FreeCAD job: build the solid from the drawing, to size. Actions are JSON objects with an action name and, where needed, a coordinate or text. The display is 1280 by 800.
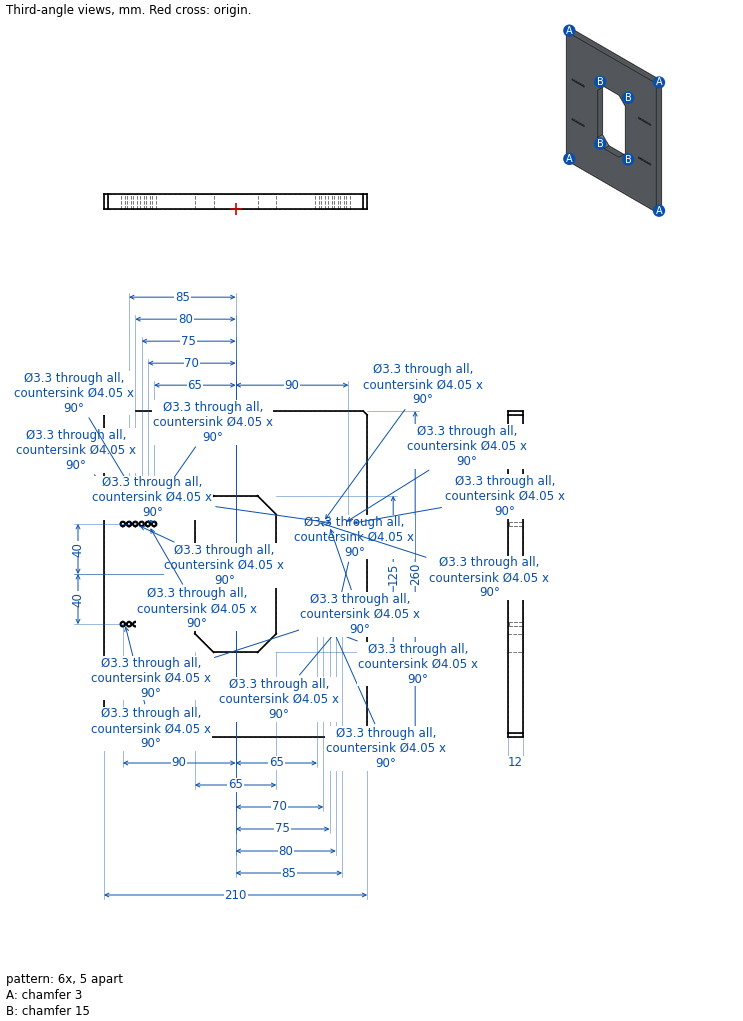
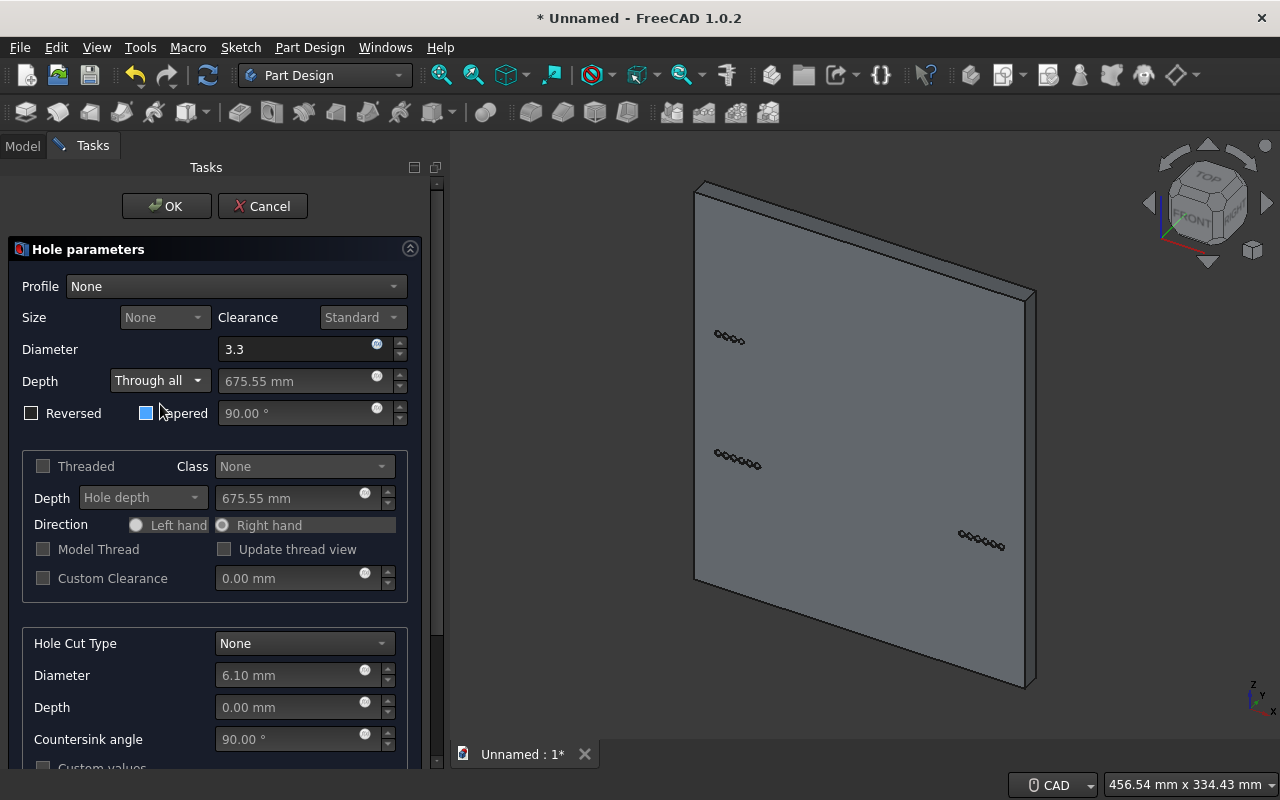
{"action": "left_click", "coordinate": [306, 644]}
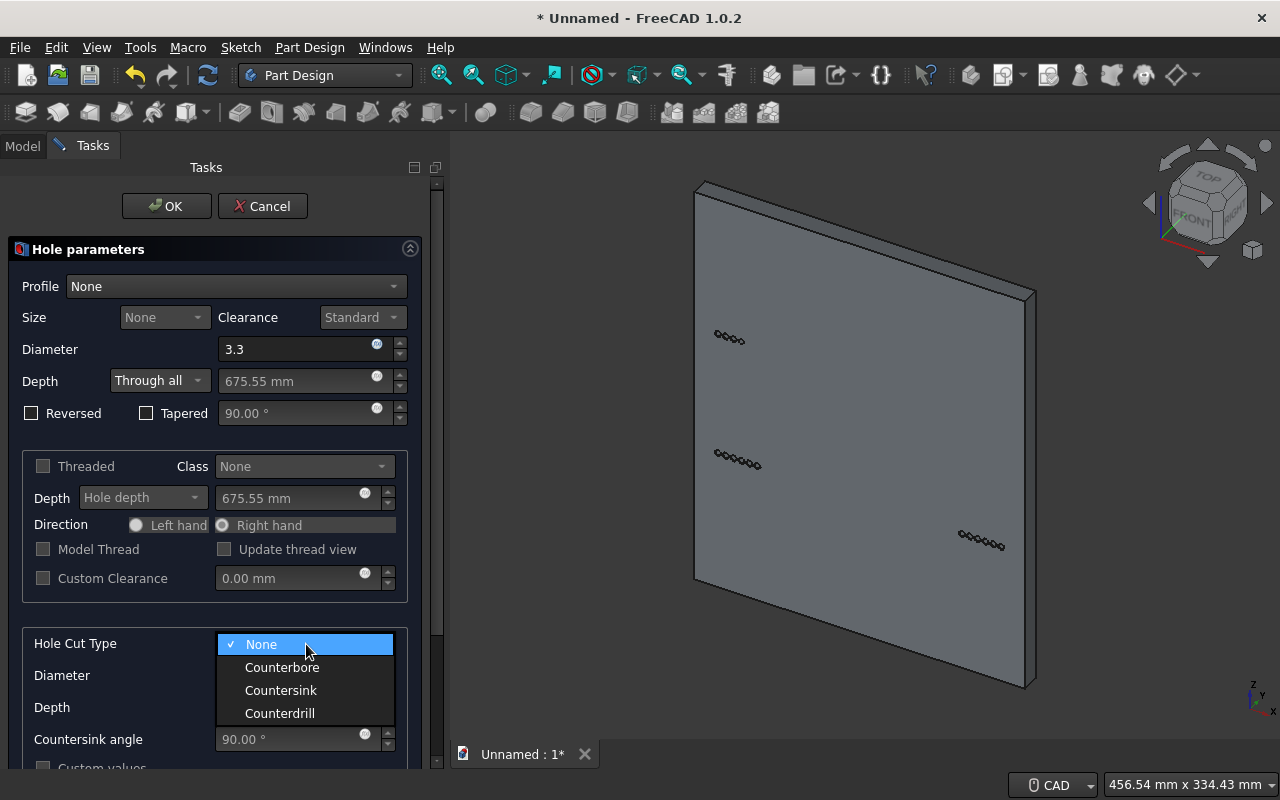
{"action": "left_click", "coordinate": [304, 690]}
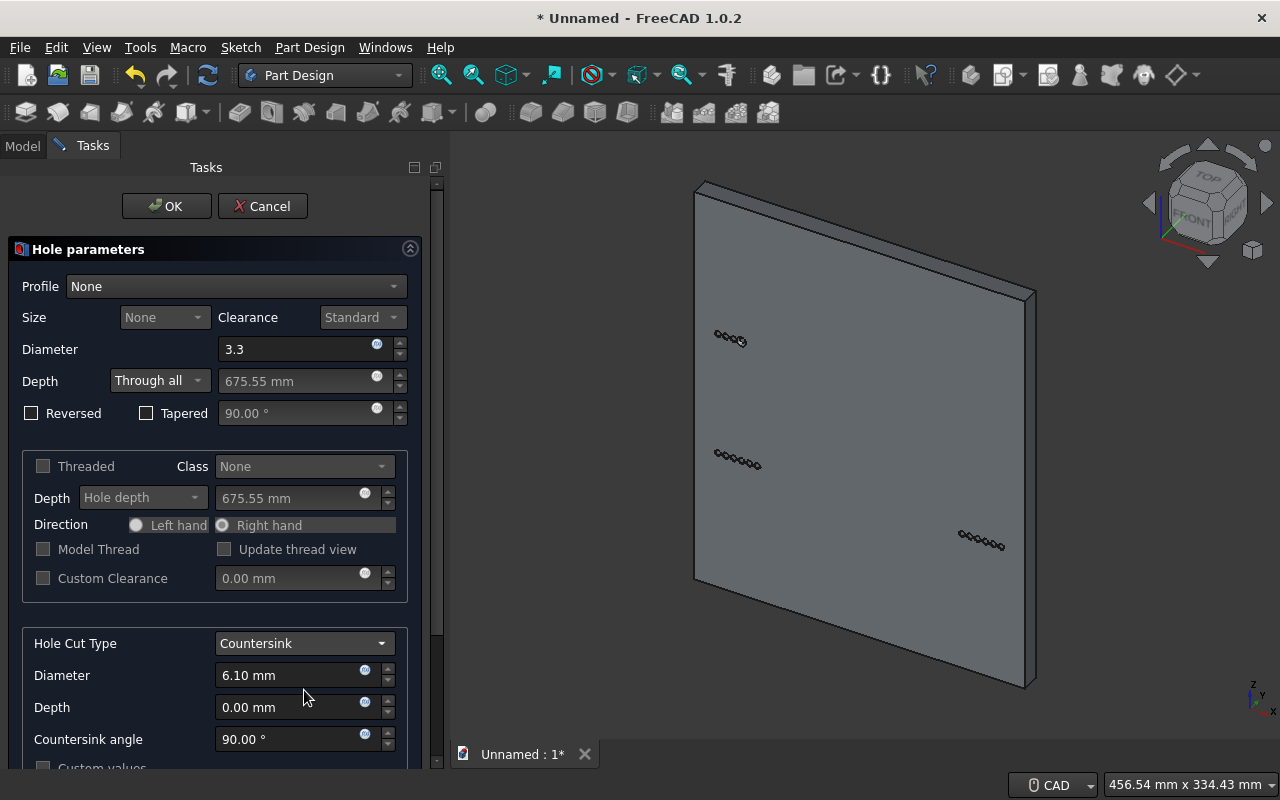
{"action": "triple_click", "coordinate": [298, 675]}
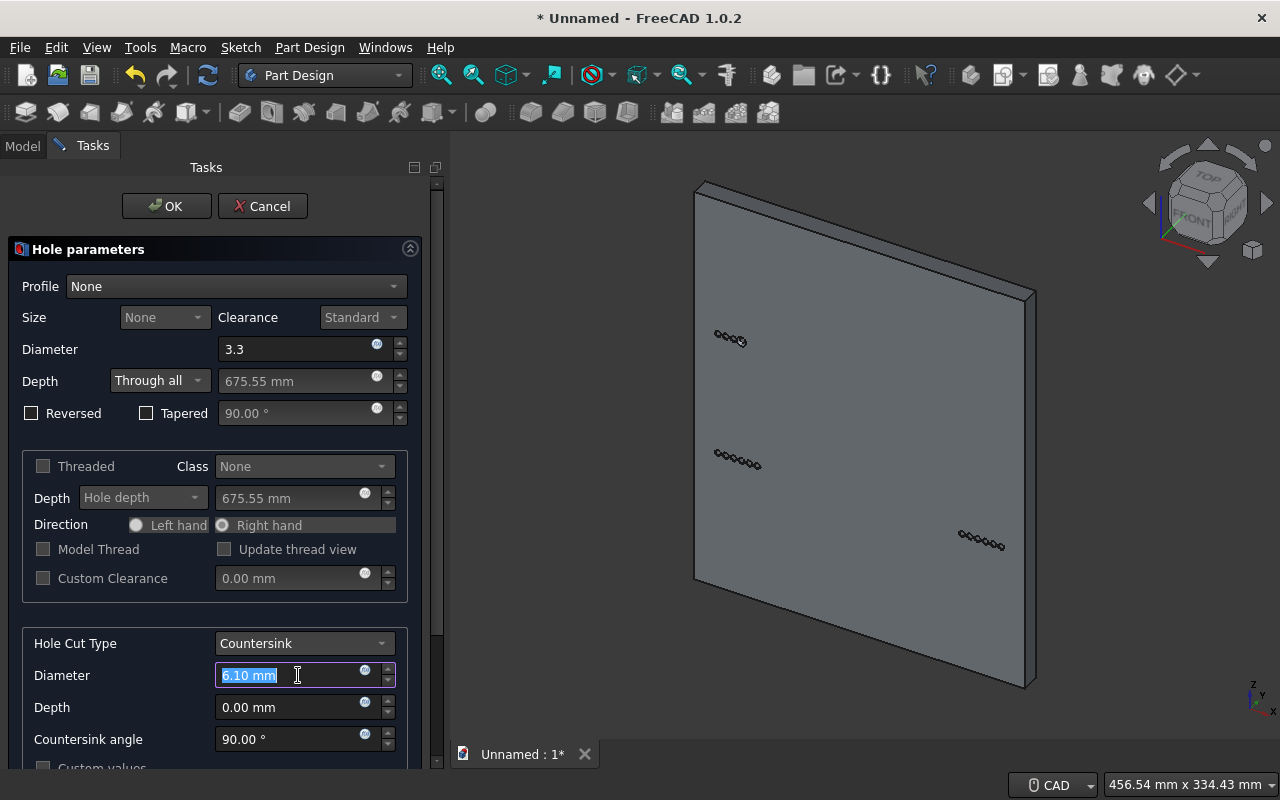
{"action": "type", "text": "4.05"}
{"action": "key", "text": "Tab"}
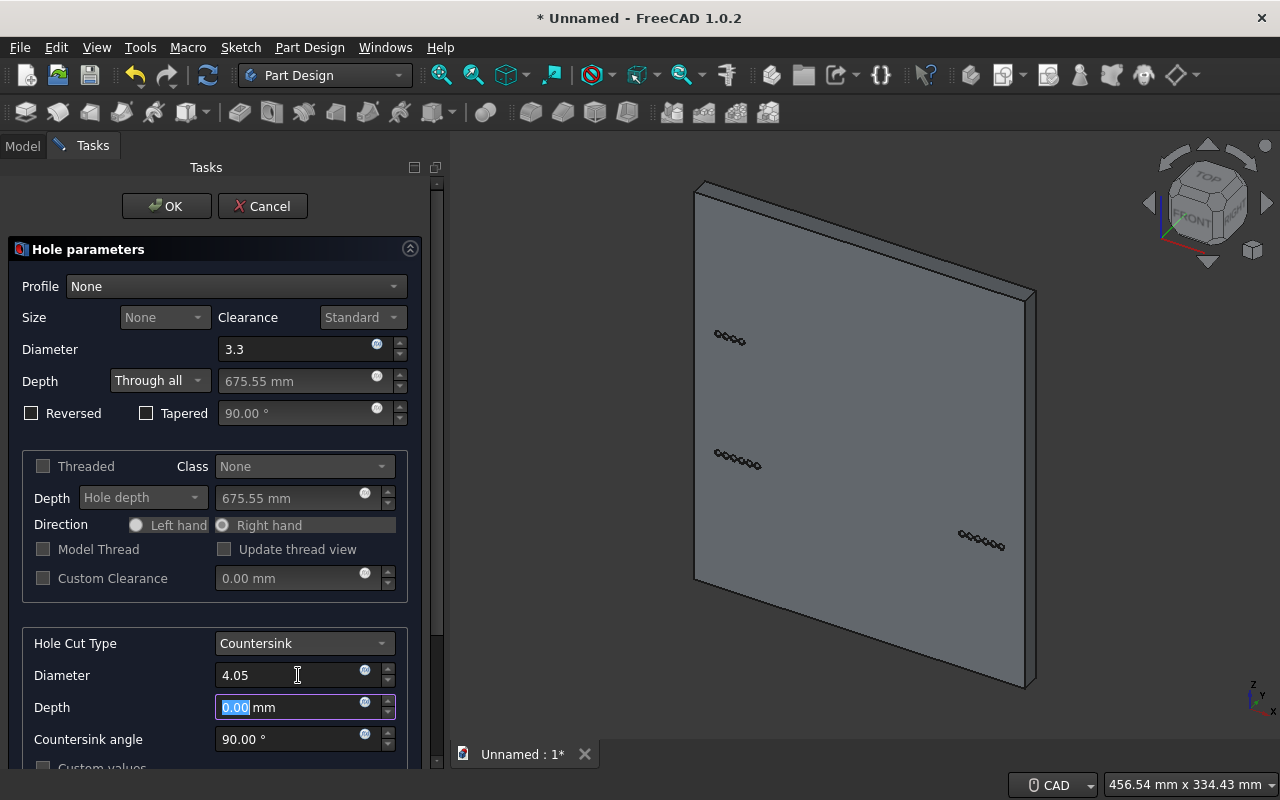
{"action": "left_click", "coordinate": [167, 206]}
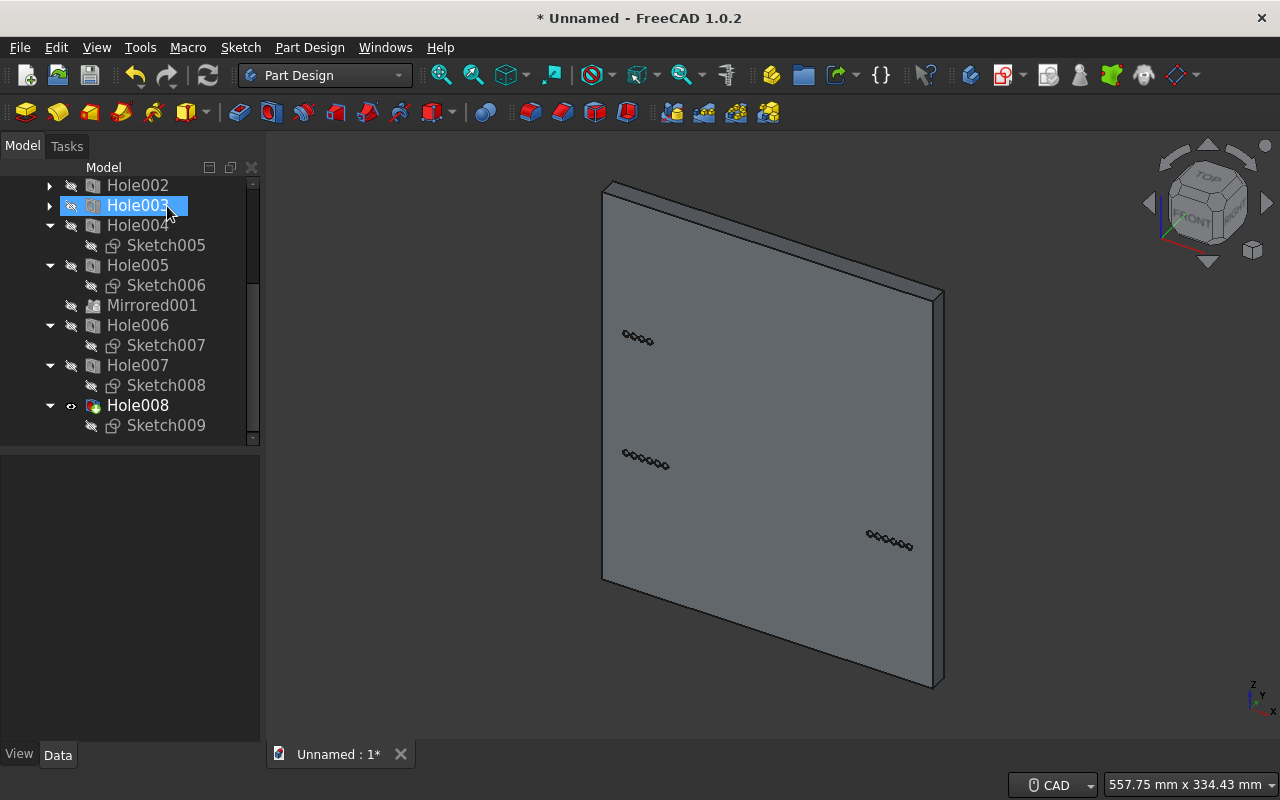
{"action": "left_click", "coordinate": [1004, 76]}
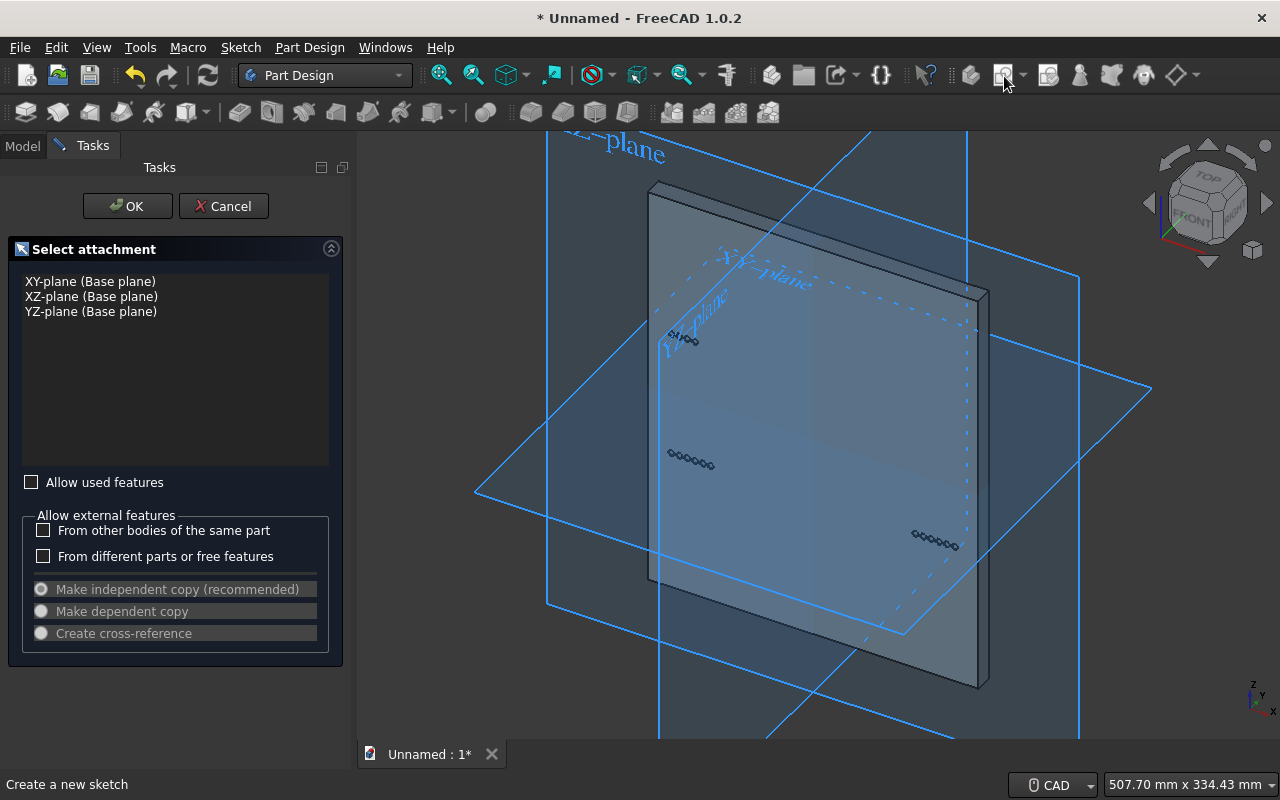
{"action": "left_click", "coordinate": [82, 296]}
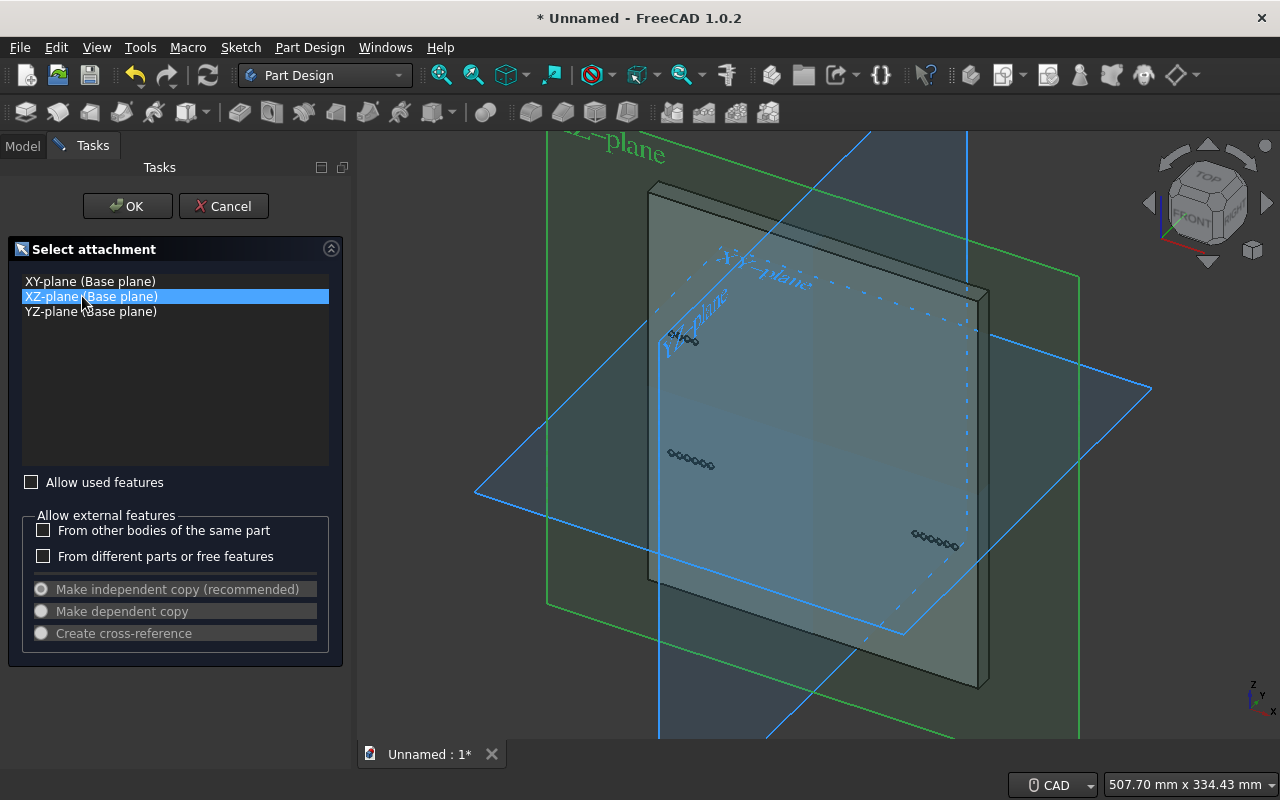
{"action": "left_click", "coordinate": [128, 206]}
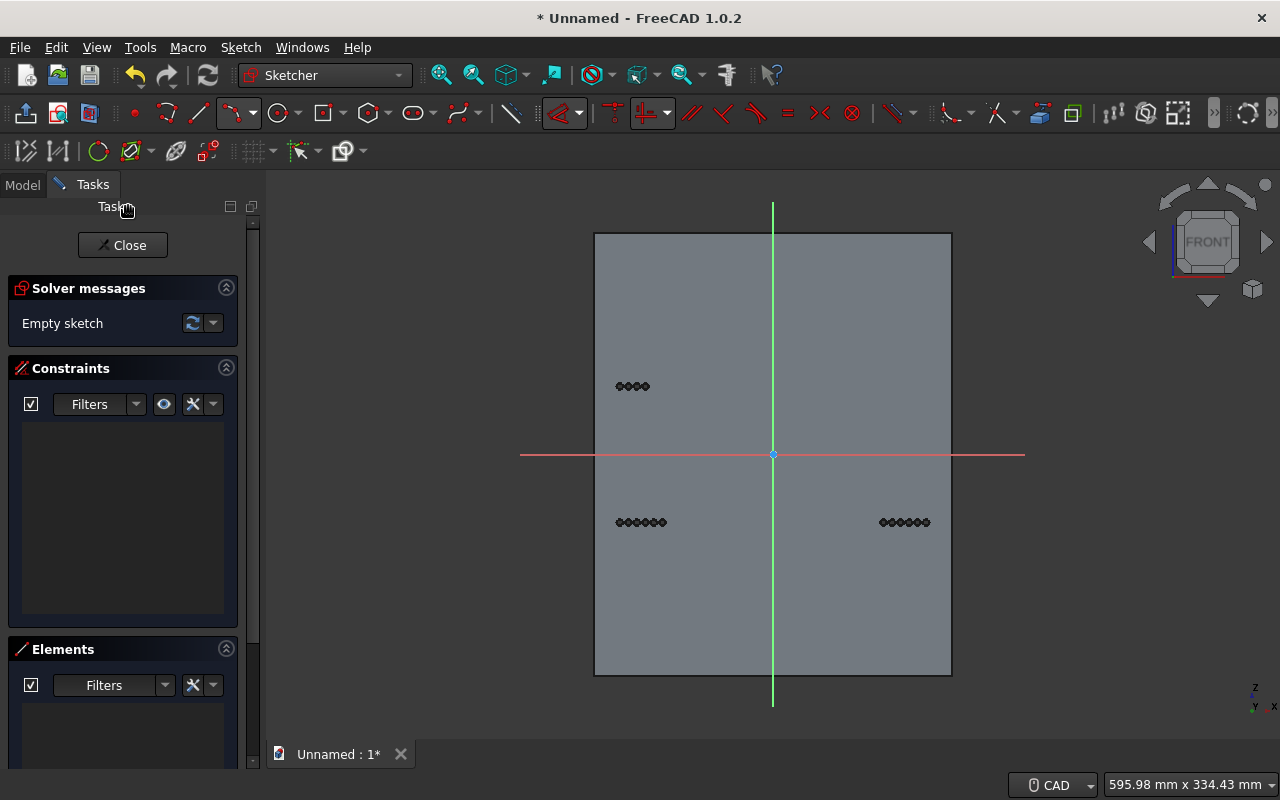
{"action": "scroll", "coordinate": [651, 383], "scroll_direction": "up", "scroll_amount": 15}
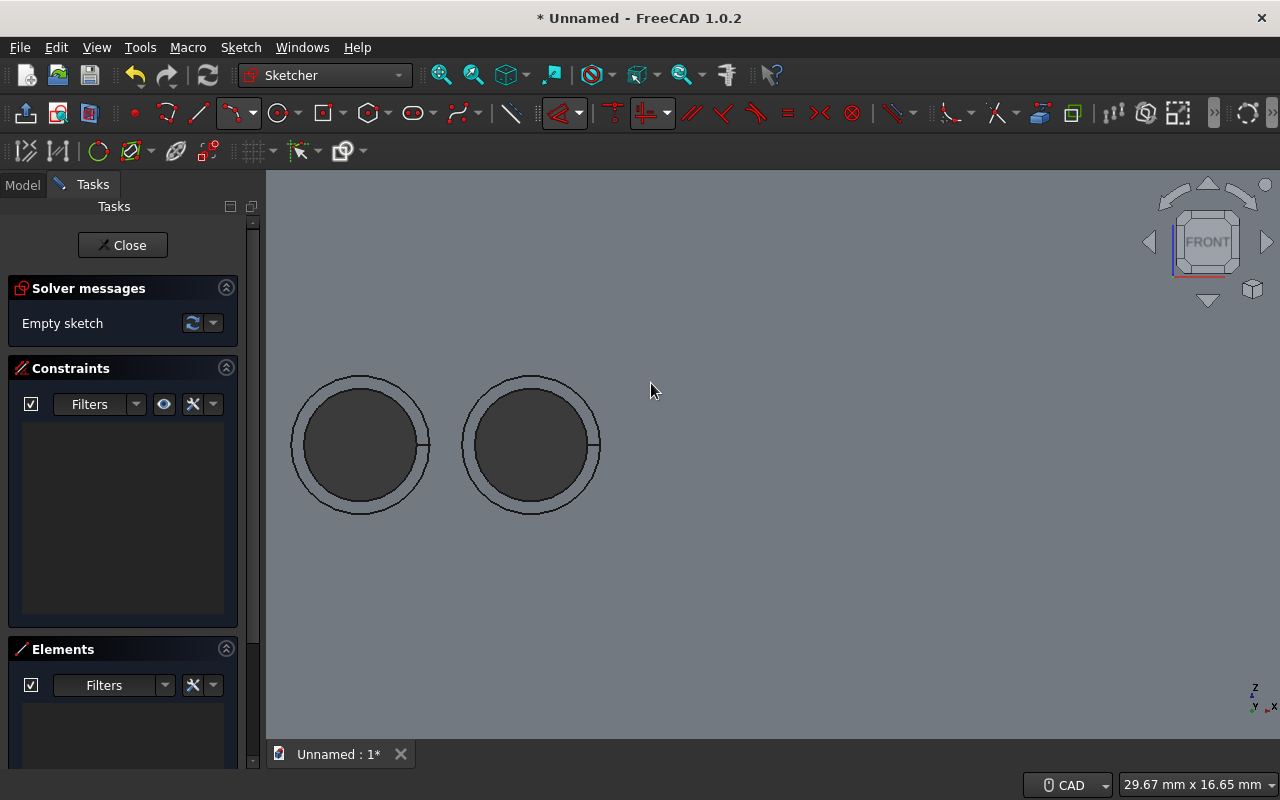
{"action": "scroll", "coordinate": [701, 441], "scroll_direction": "up", "scroll_amount": 6}